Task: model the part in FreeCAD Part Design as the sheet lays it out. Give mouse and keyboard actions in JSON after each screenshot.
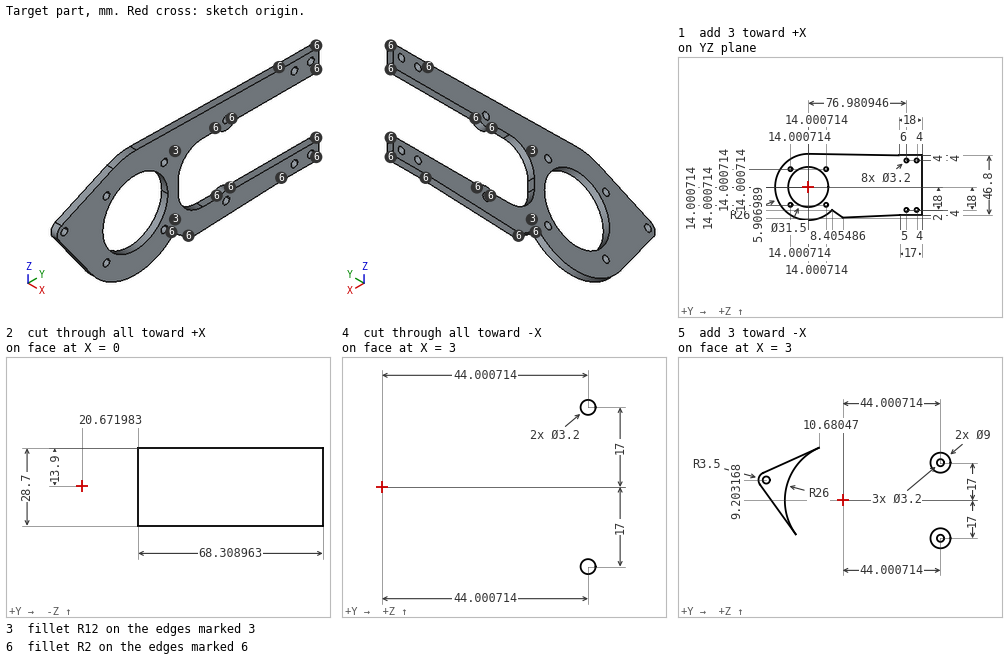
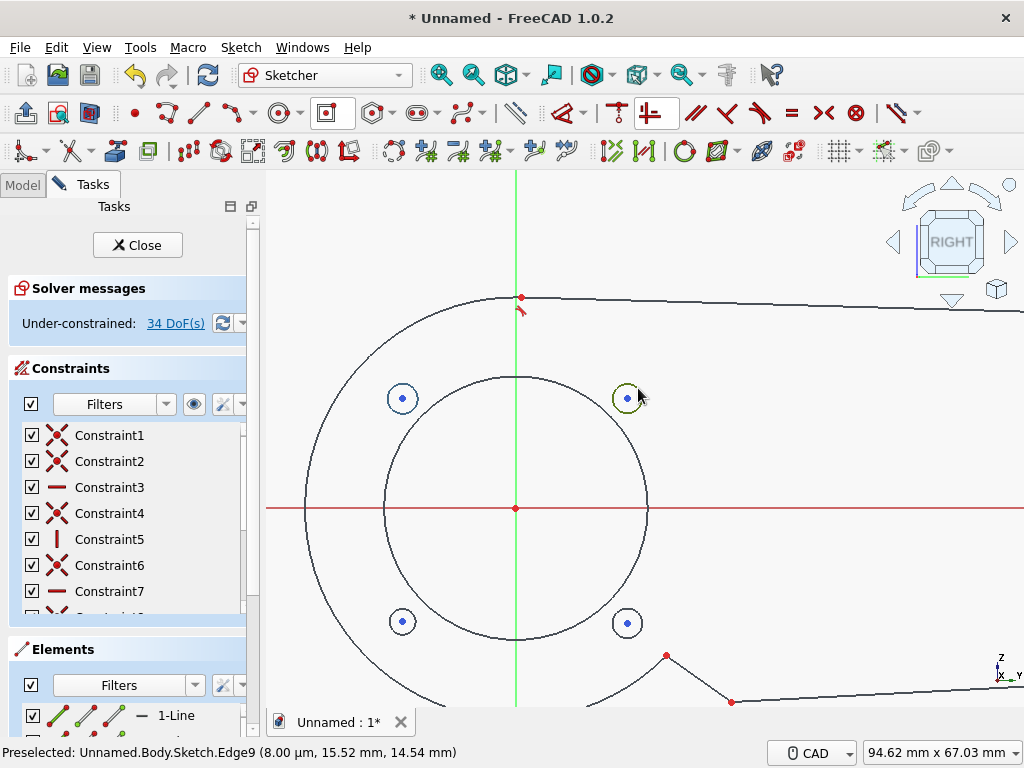
{"action": "left_click", "coordinate": [412, 613]}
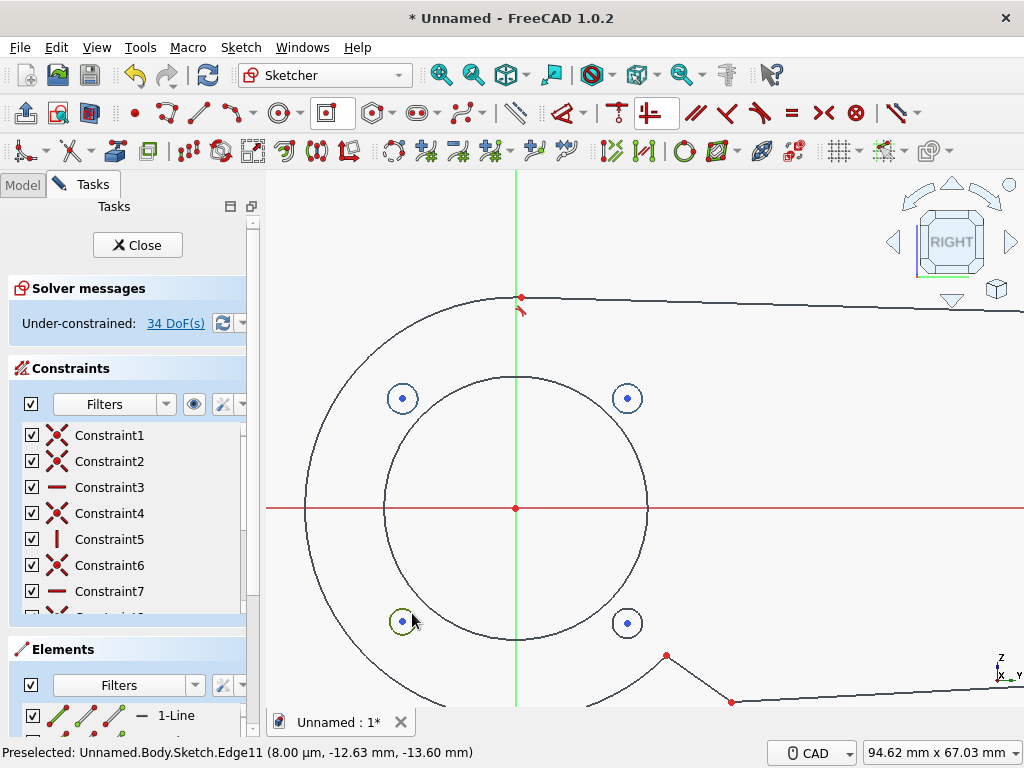
{"action": "left_click", "coordinate": [638, 613]}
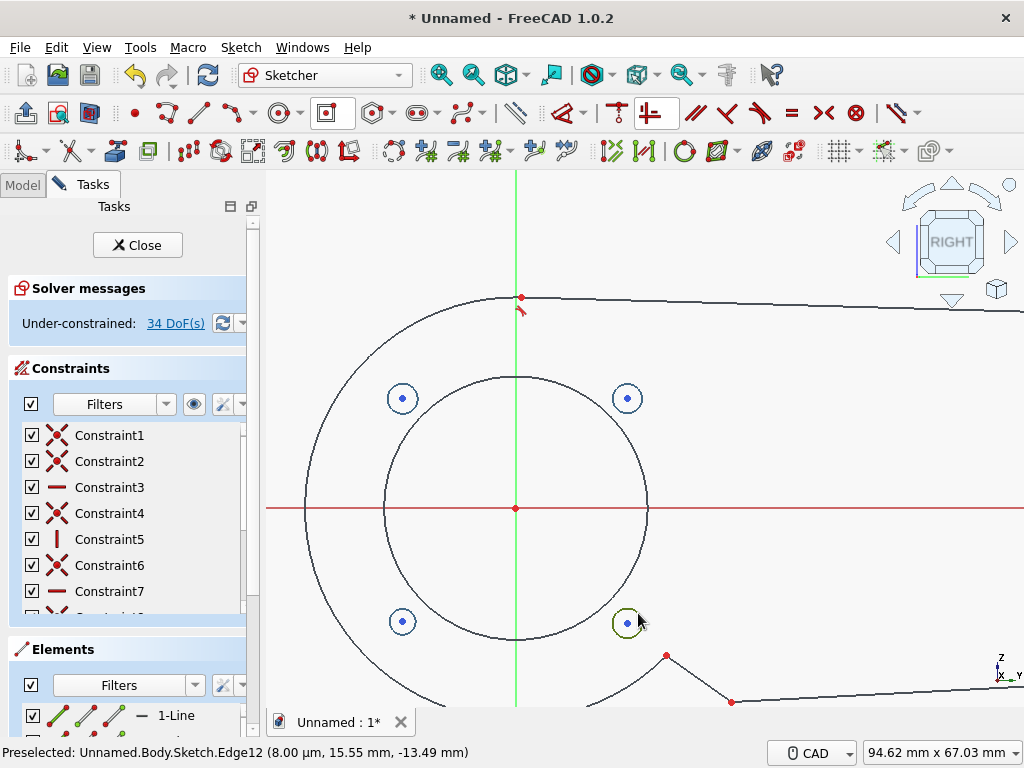
{"action": "scroll", "coordinate": [414, 388], "scroll_direction": "down", "scroll_amount": 4}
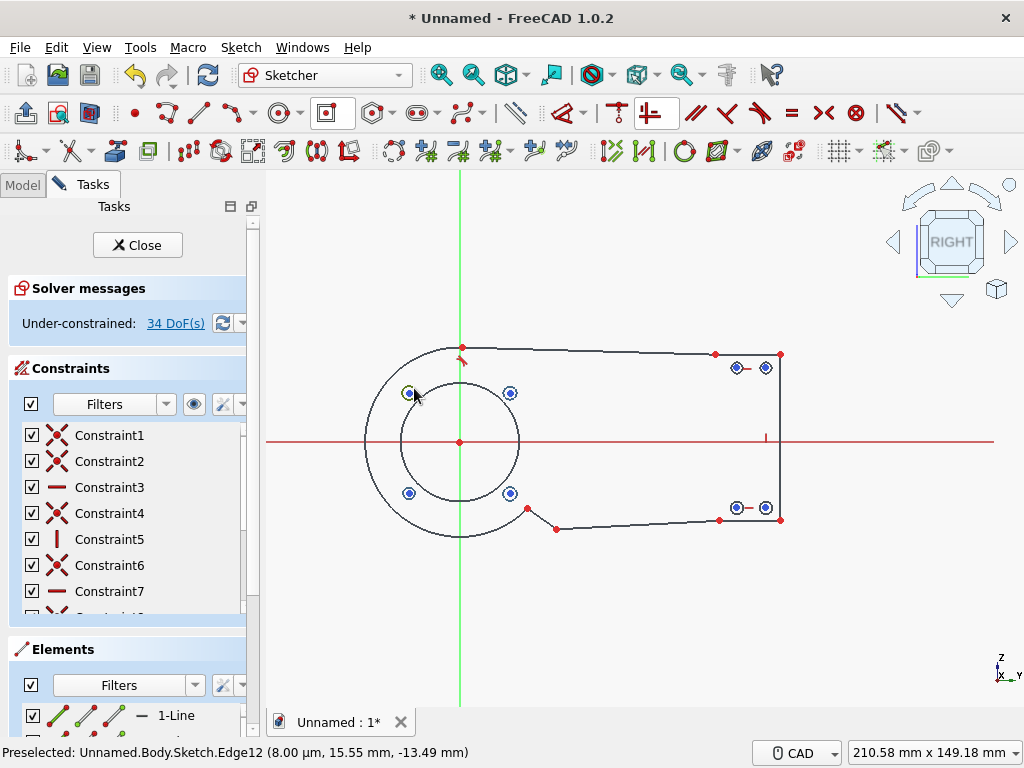
{"action": "scroll", "coordinate": [741, 364], "scroll_direction": "up", "scroll_amount": 5}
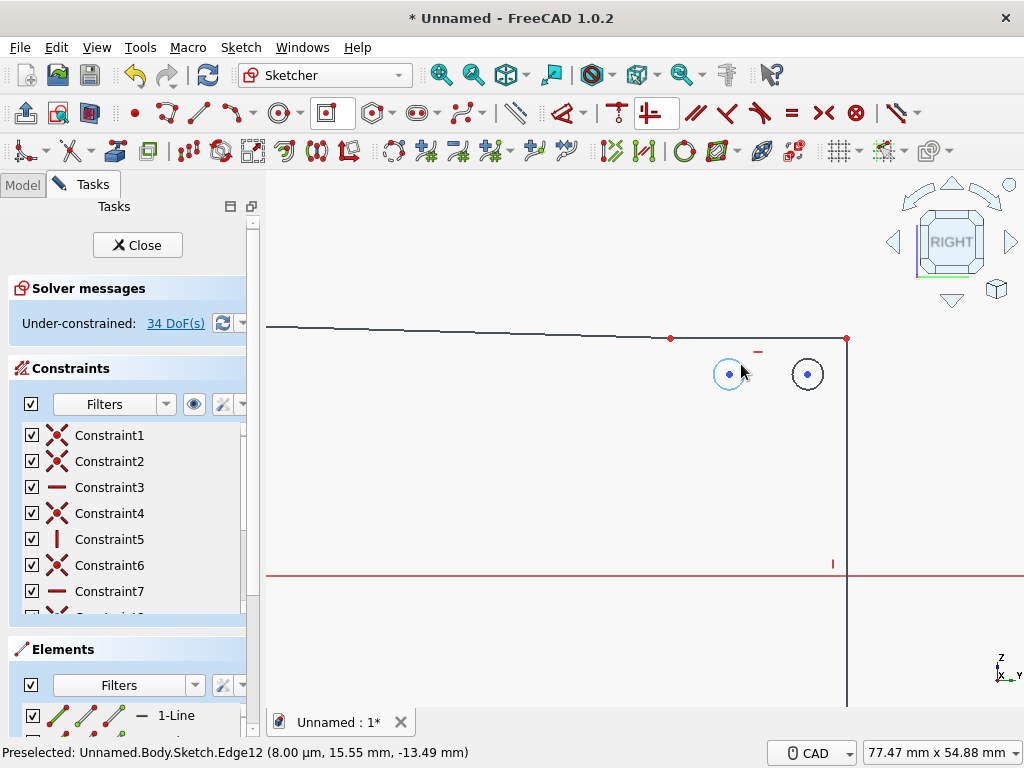
{"action": "left_click", "coordinate": [740, 363]}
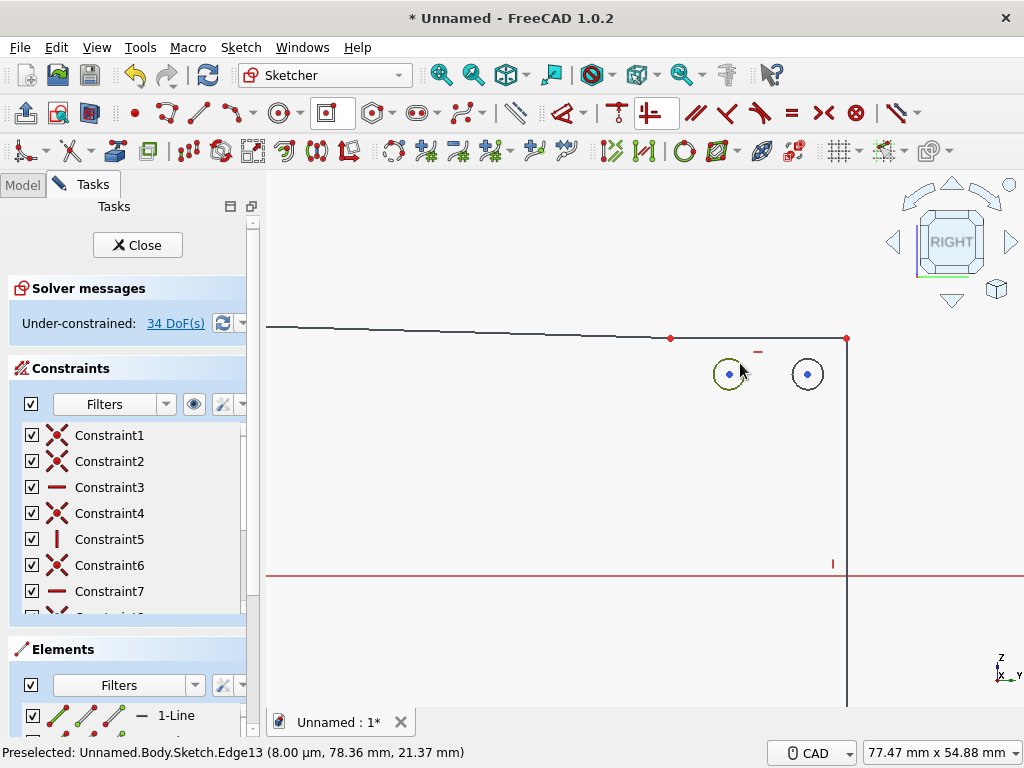
{"action": "left_click", "coordinate": [819, 363]}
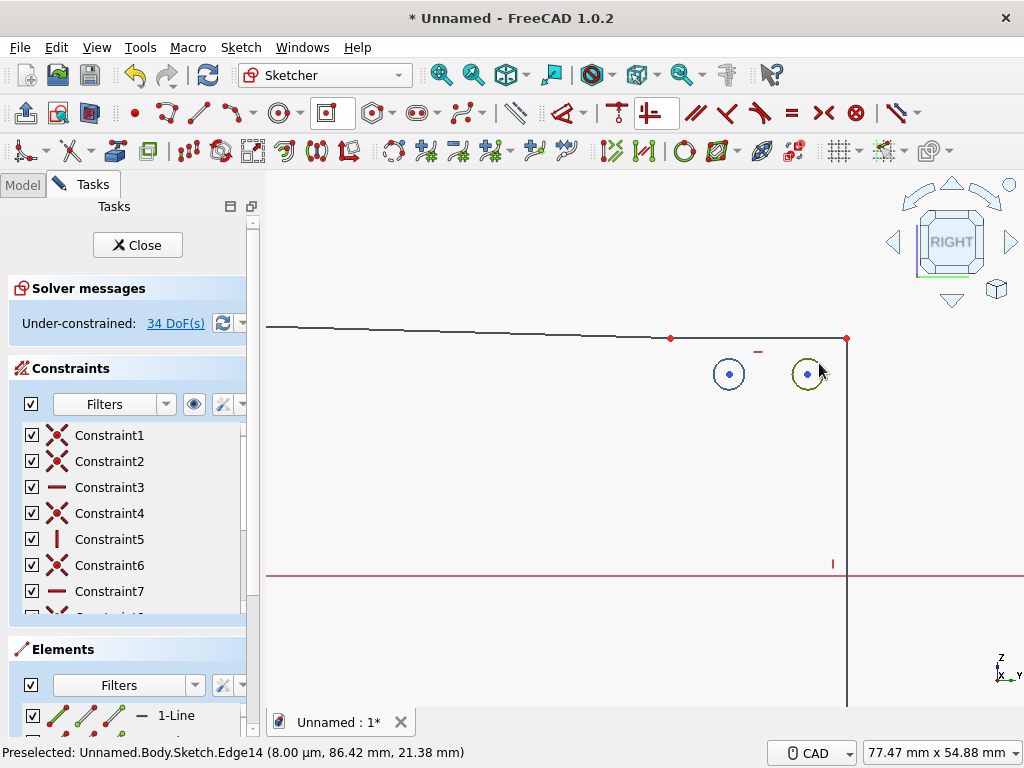
{"action": "scroll", "coordinate": [741, 364], "scroll_direction": "down", "scroll_amount": 5}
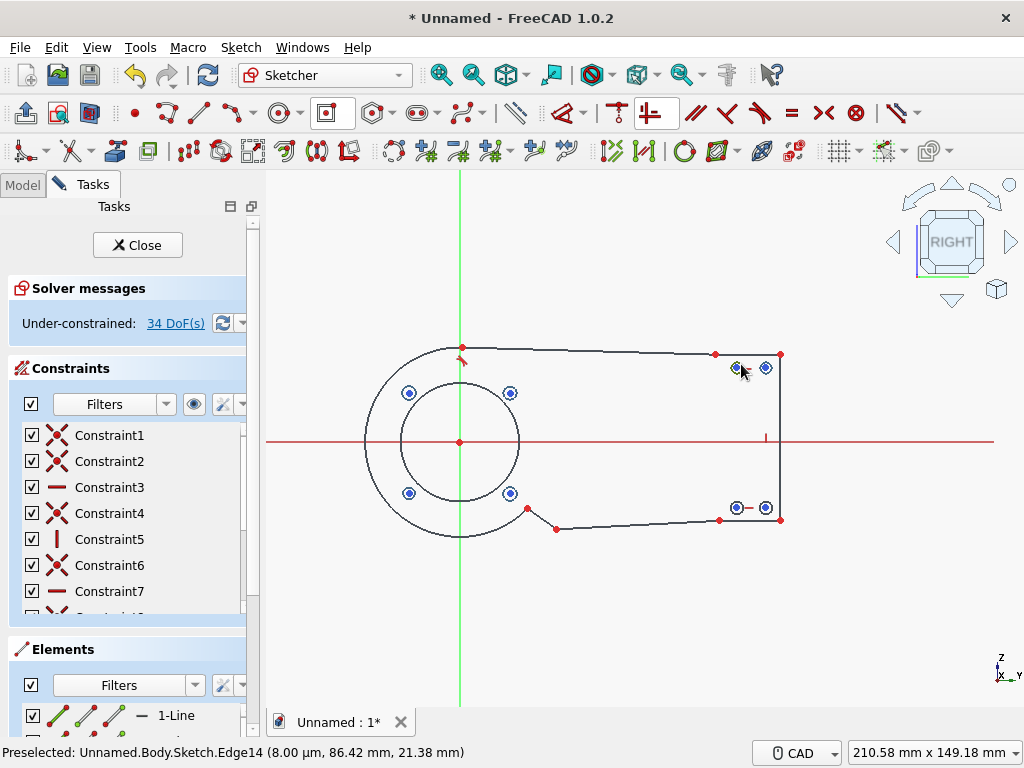
{"action": "scroll", "coordinate": [742, 503], "scroll_direction": "up", "scroll_amount": 4}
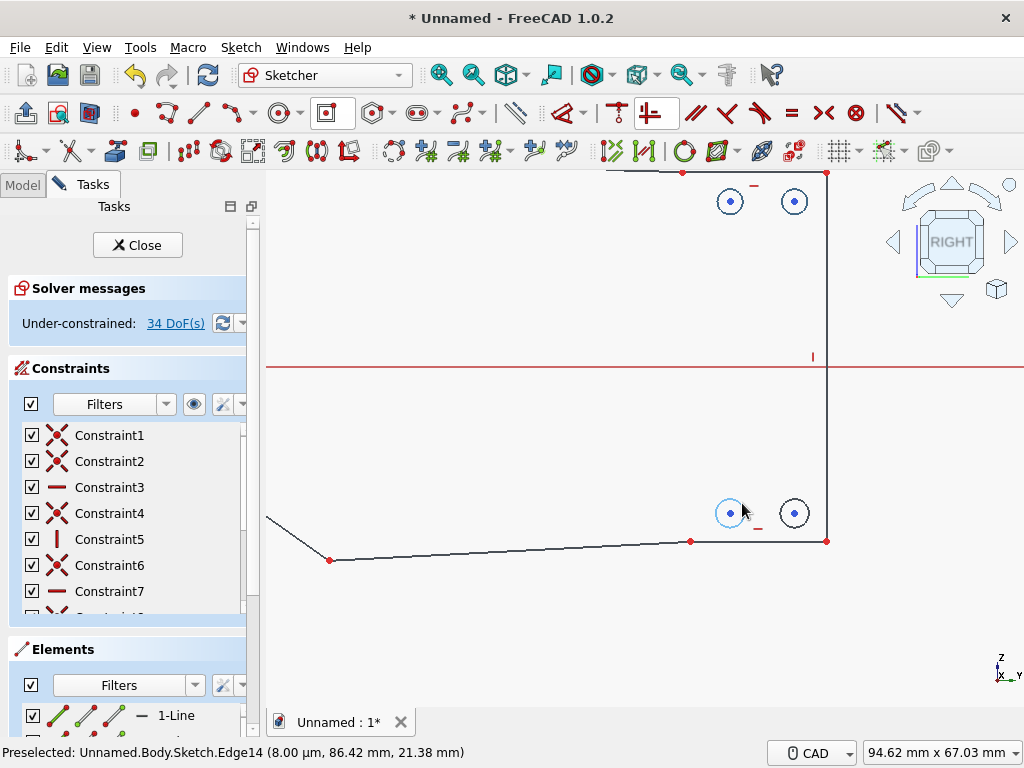
{"action": "left_click", "coordinate": [740, 503]}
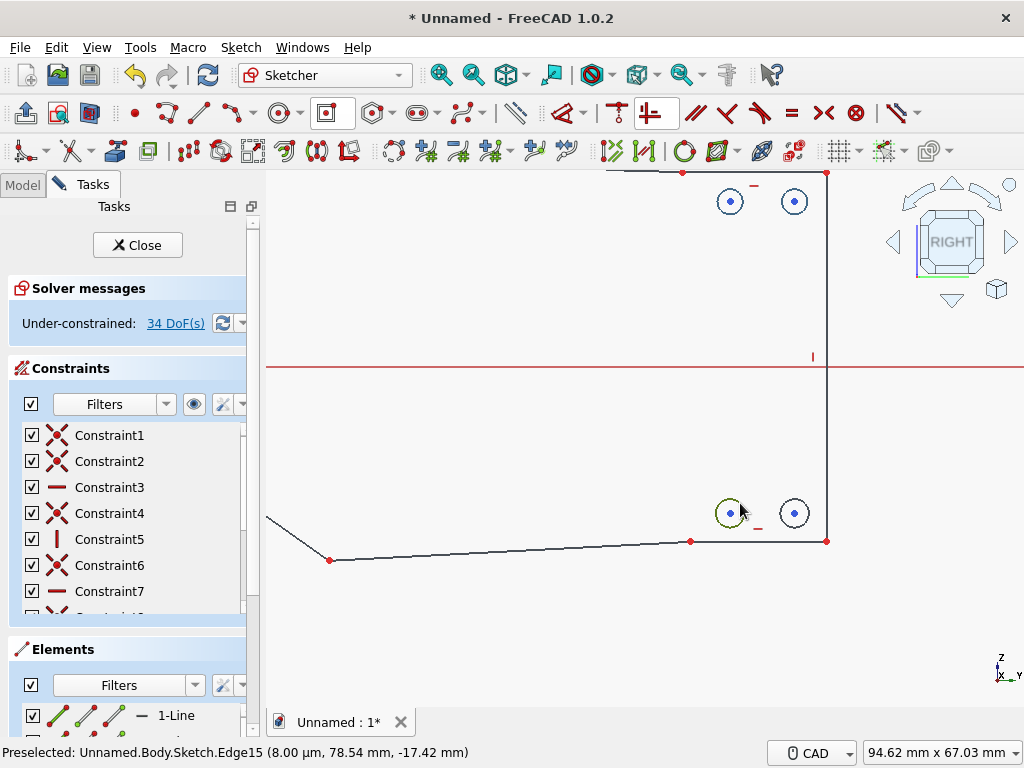
{"action": "left_click", "coordinate": [805, 503]}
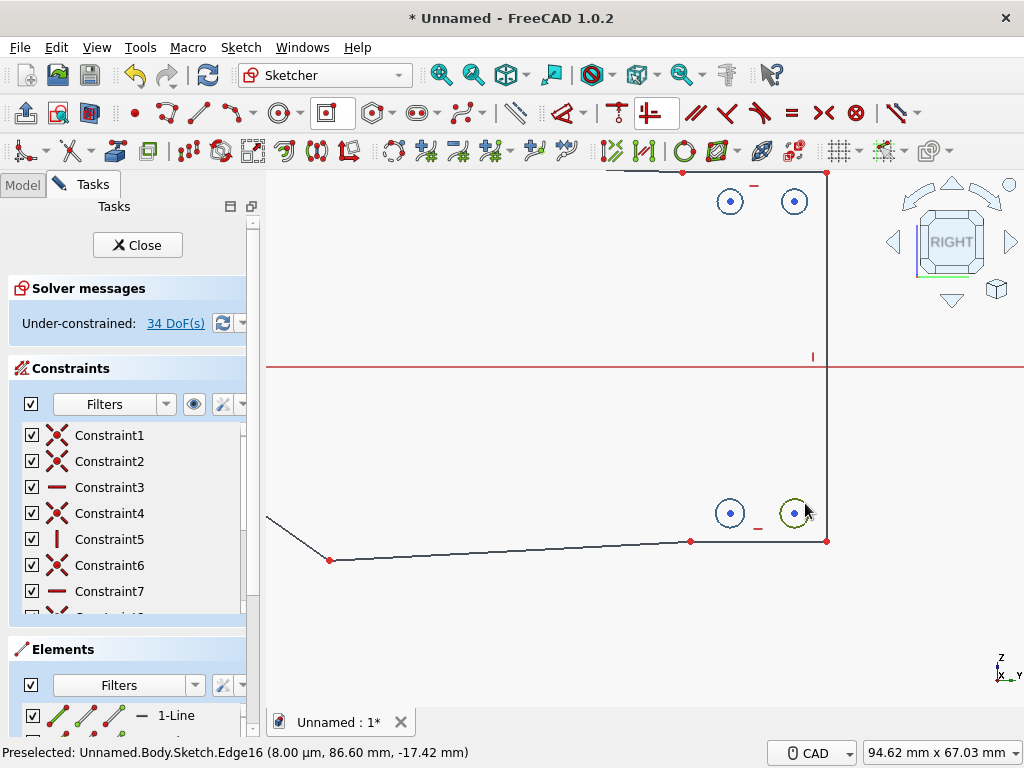
{"action": "left_click", "coordinate": [792, 114]}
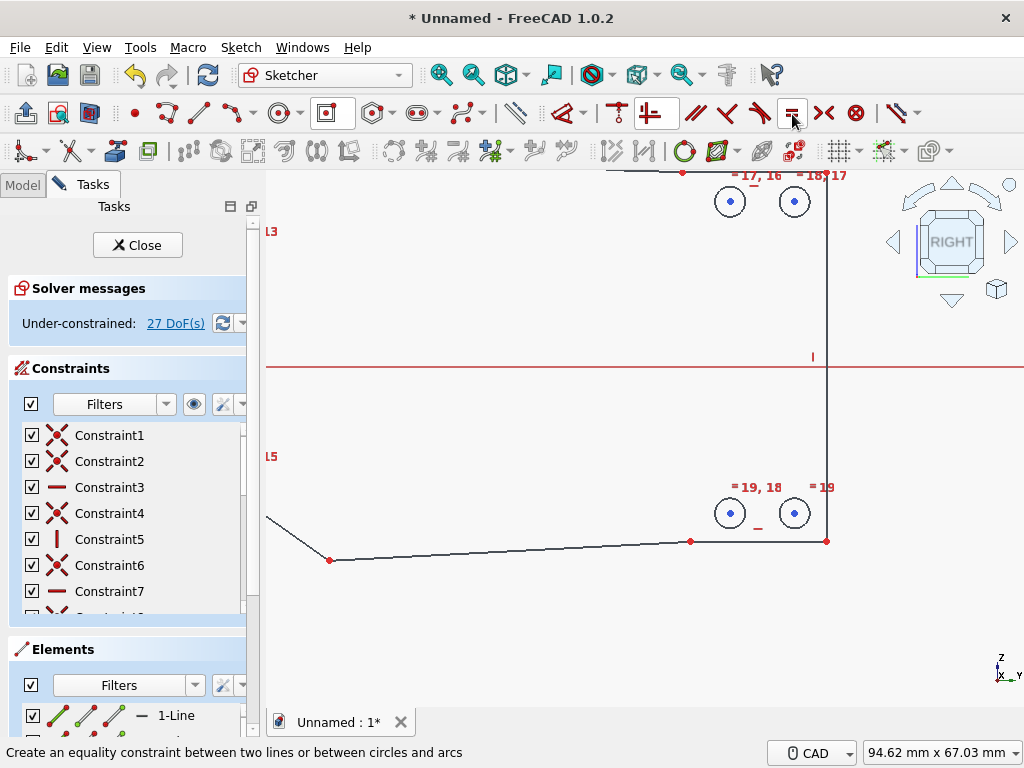
{"action": "scroll", "coordinate": [742, 503], "scroll_direction": "down", "scroll_amount": 4}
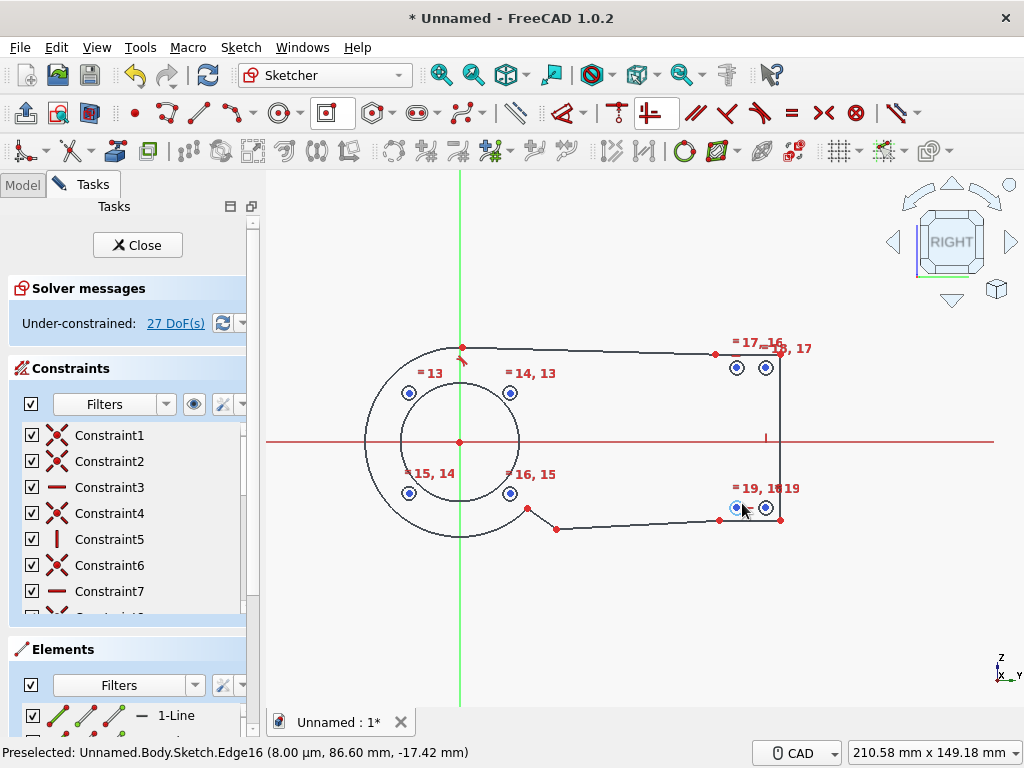
{"action": "left_click", "coordinate": [373, 404]}